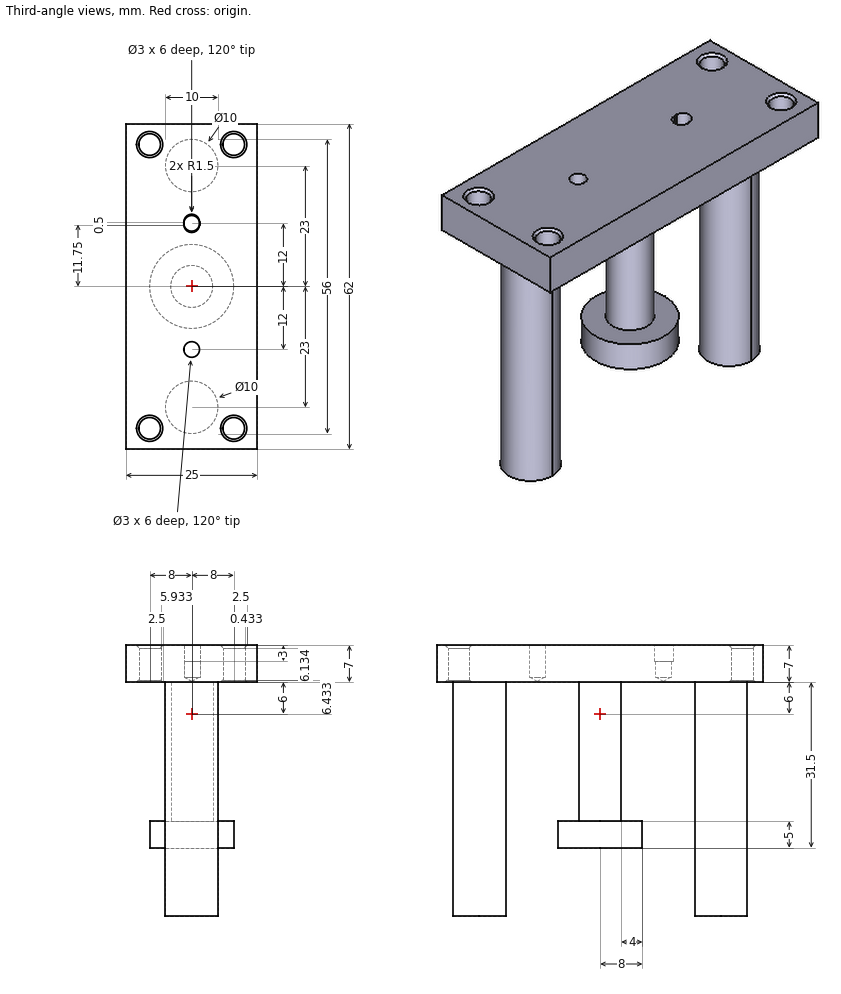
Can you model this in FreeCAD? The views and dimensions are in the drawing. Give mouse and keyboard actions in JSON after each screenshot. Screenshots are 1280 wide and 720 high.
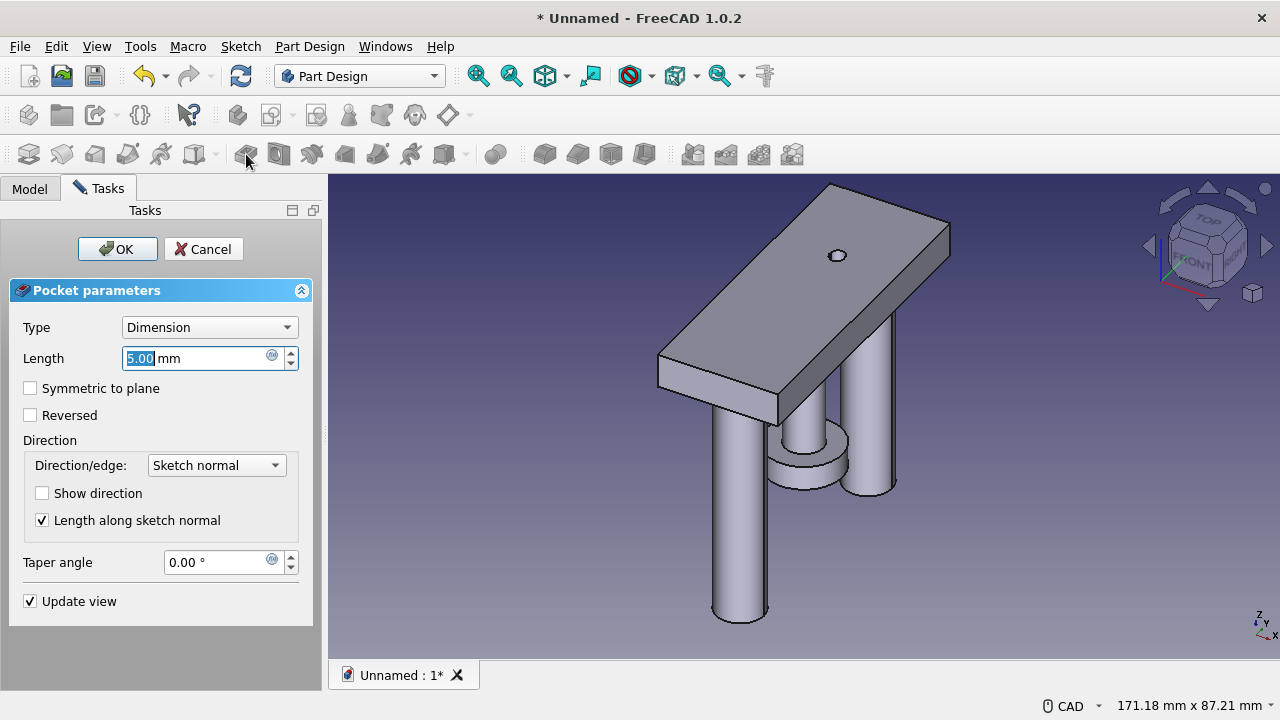
{"action": "type", "text": "3"}
{"action": "key", "text": "Tab"}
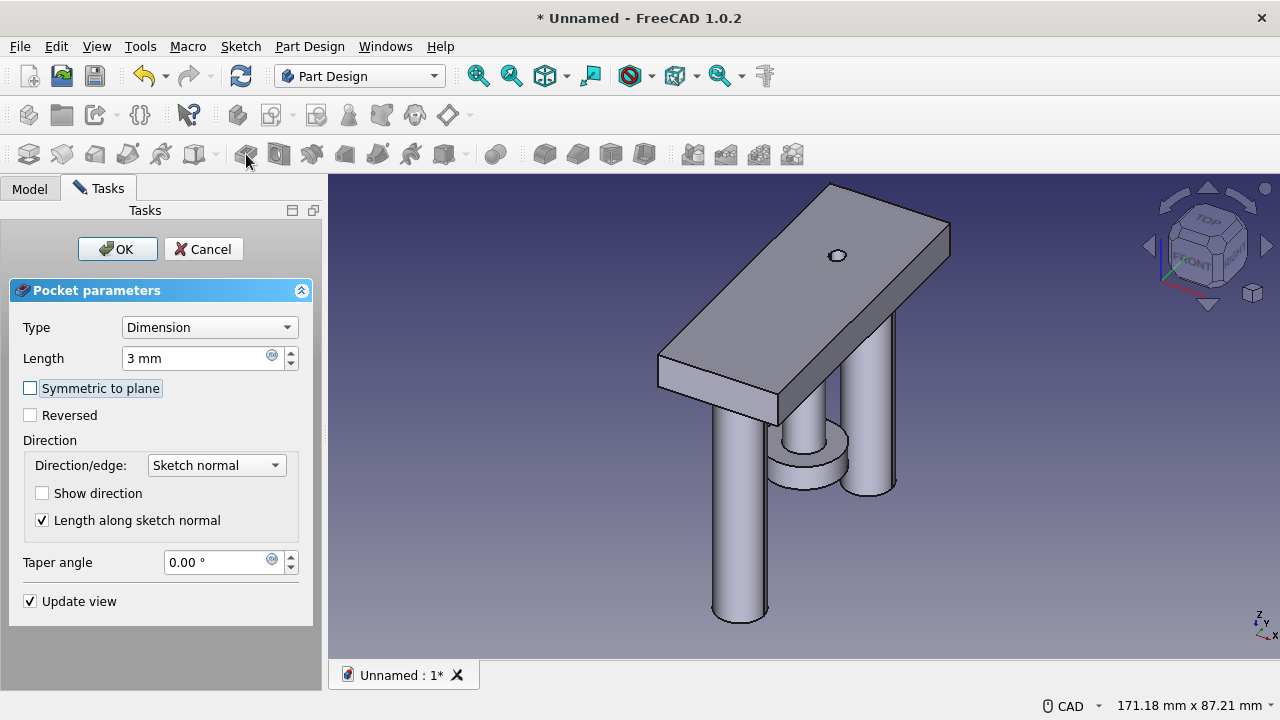
{"action": "left_click", "coordinate": [118, 249]}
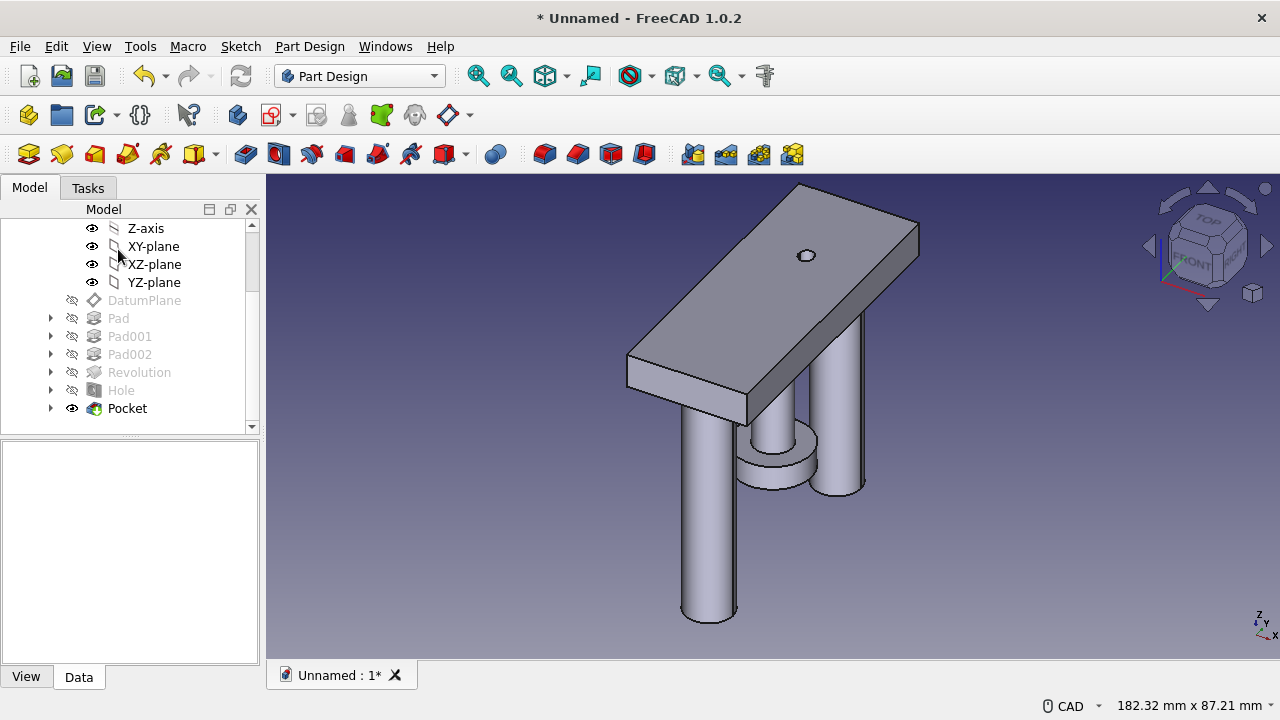
{"action": "left_click", "coordinate": [748, 312]}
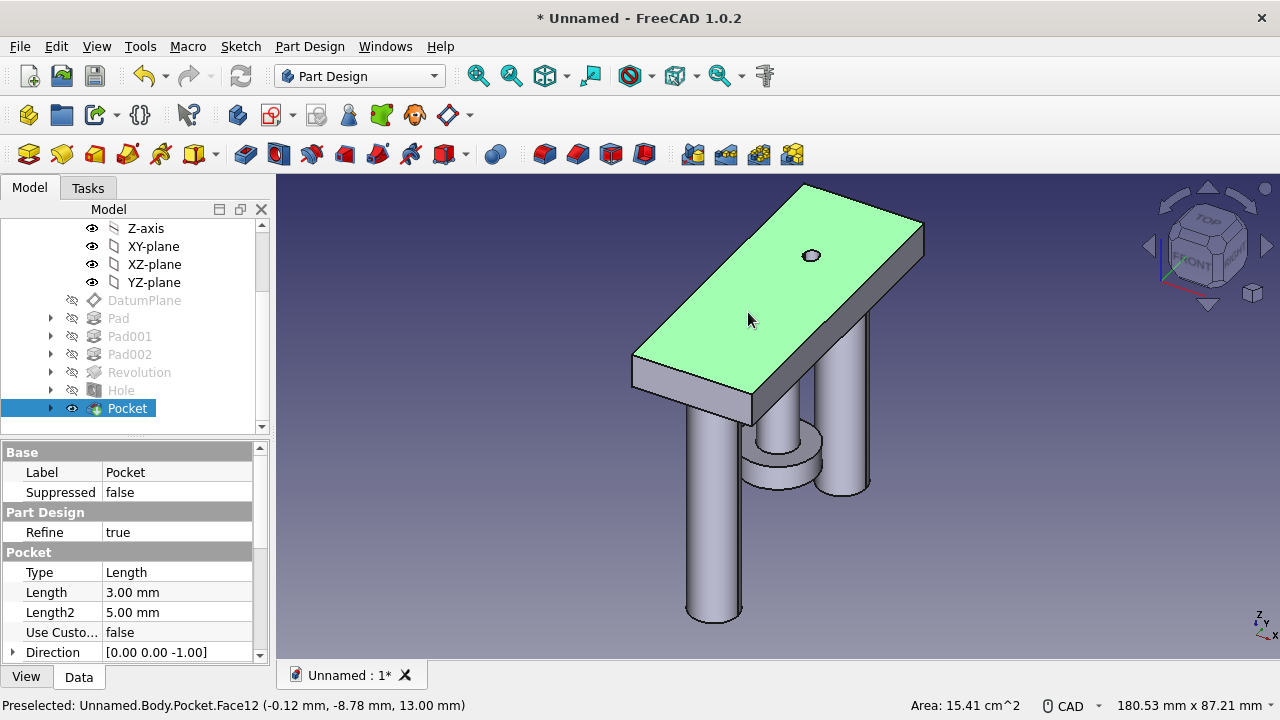
{"action": "left_click", "coordinate": [270, 116]}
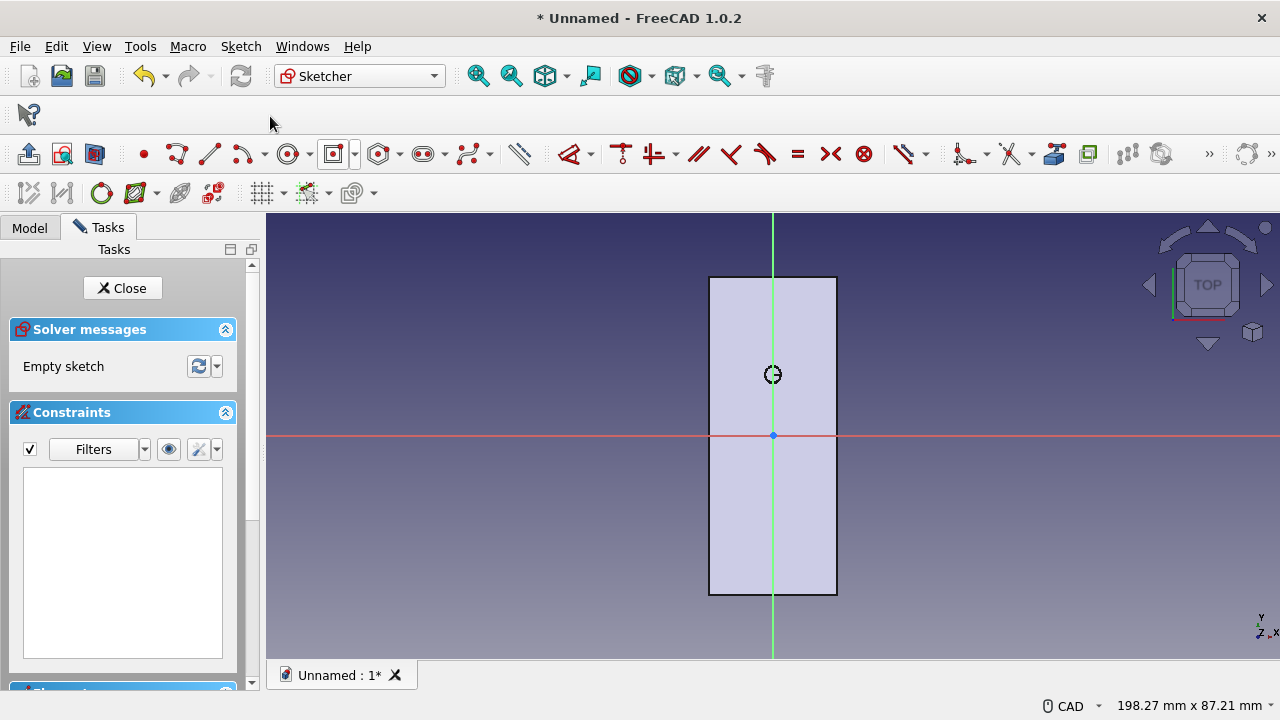
{"action": "scroll", "coordinate": [777, 501], "scroll_direction": "up", "scroll_amount": 14}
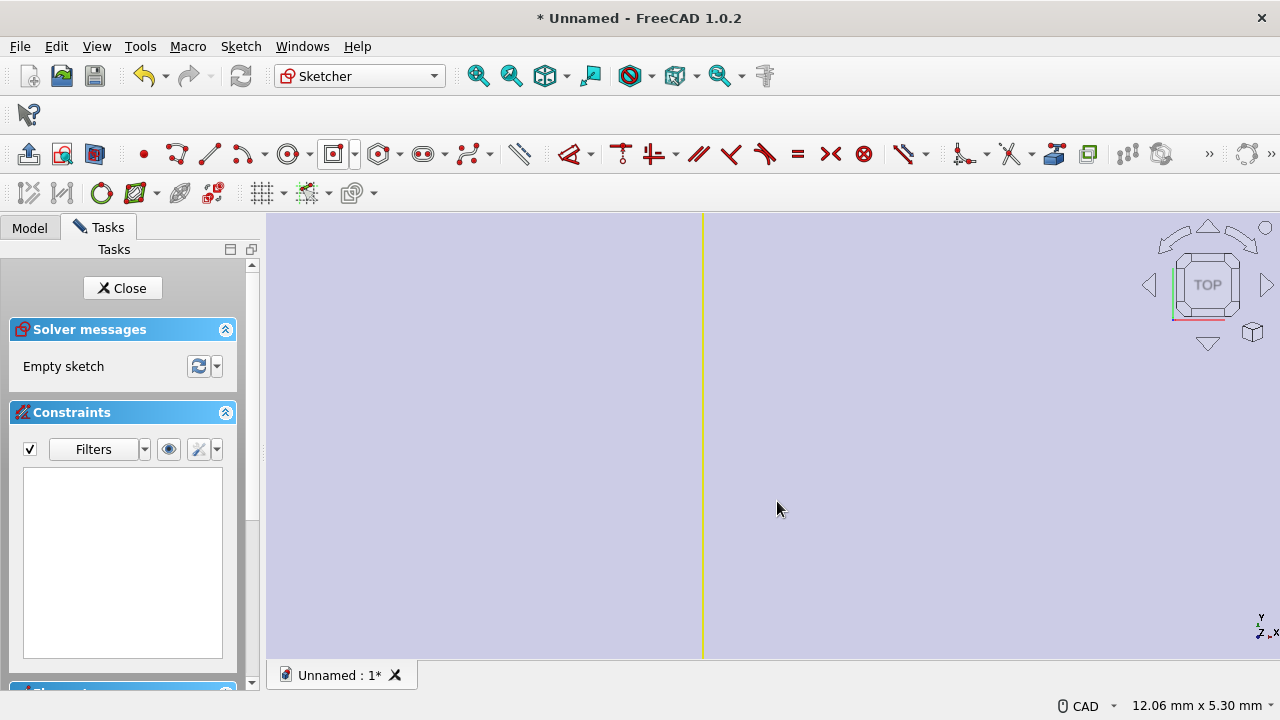
{"action": "left_click", "coordinate": [288, 154]}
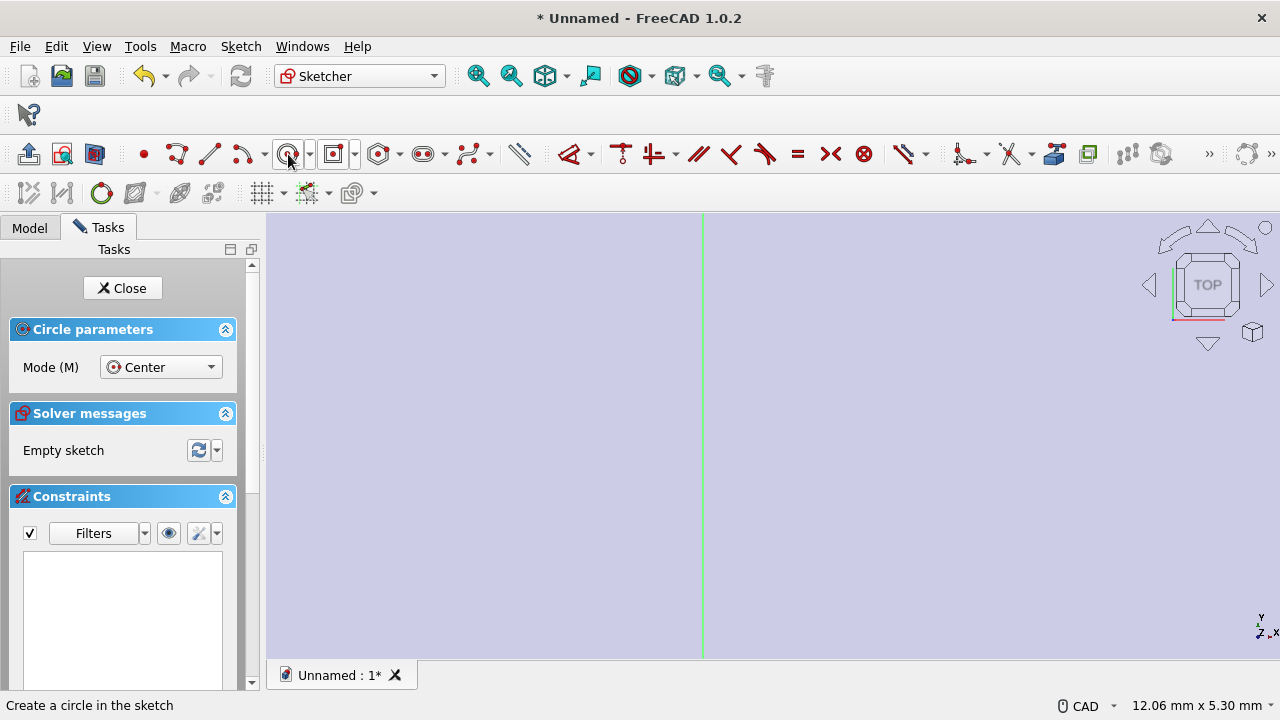
{"action": "left_click", "coordinate": [703, 431]}
{"action": "left_click", "coordinate": [793, 342]}
{"action": "key", "text": "Escape"}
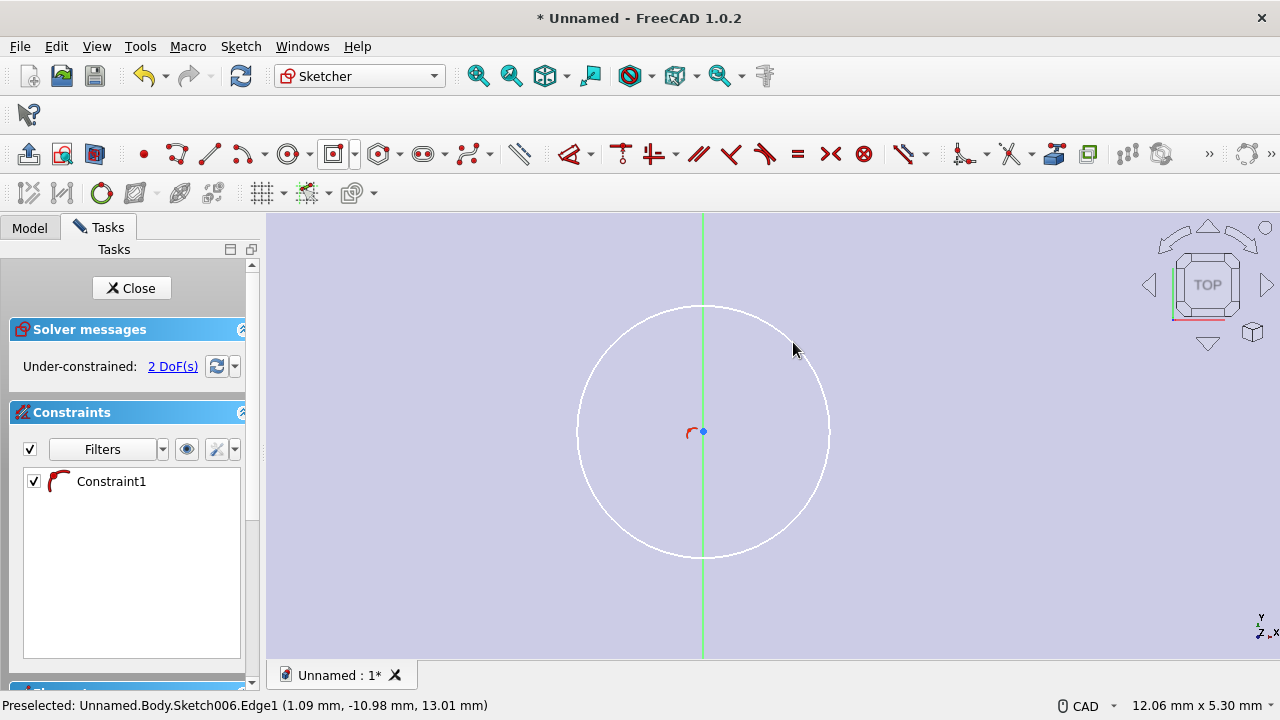
{"action": "left_click", "coordinate": [568, 154]}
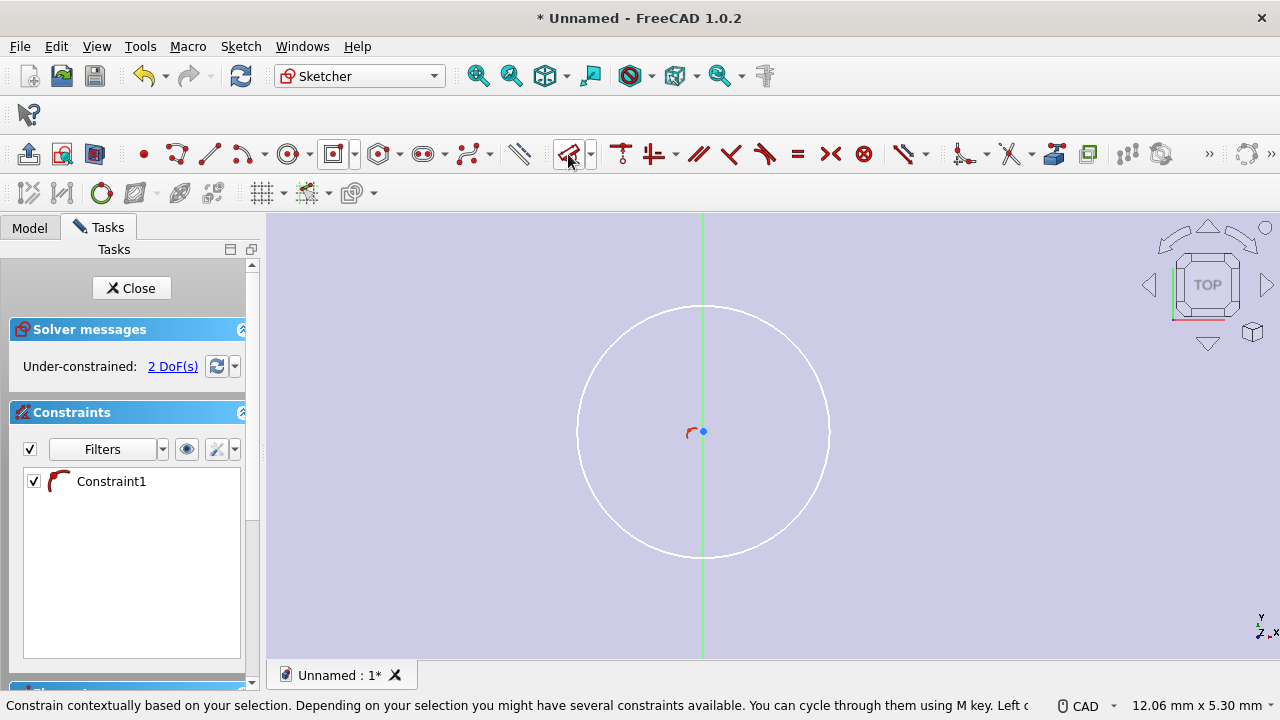
{"action": "left_click", "coordinate": [792, 342]}
{"action": "left_click", "coordinate": [814, 319]}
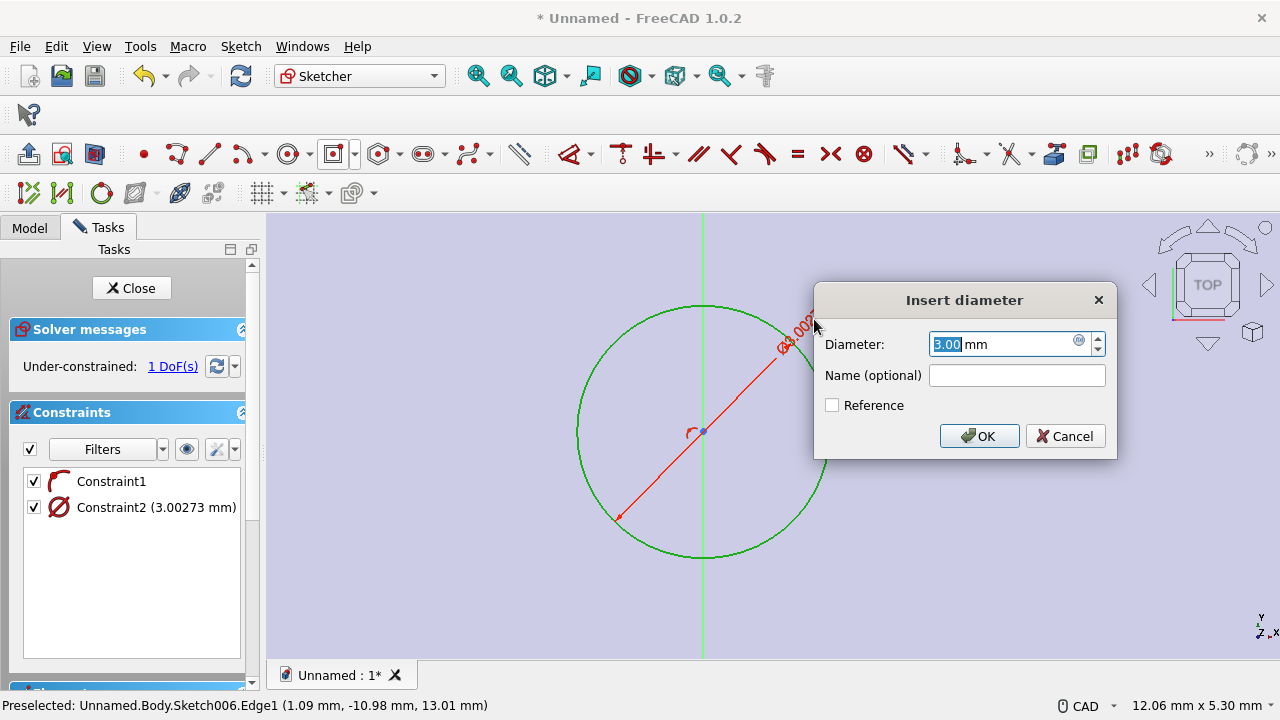
{"action": "type", "text": "3"}
{"action": "key", "text": "Return"}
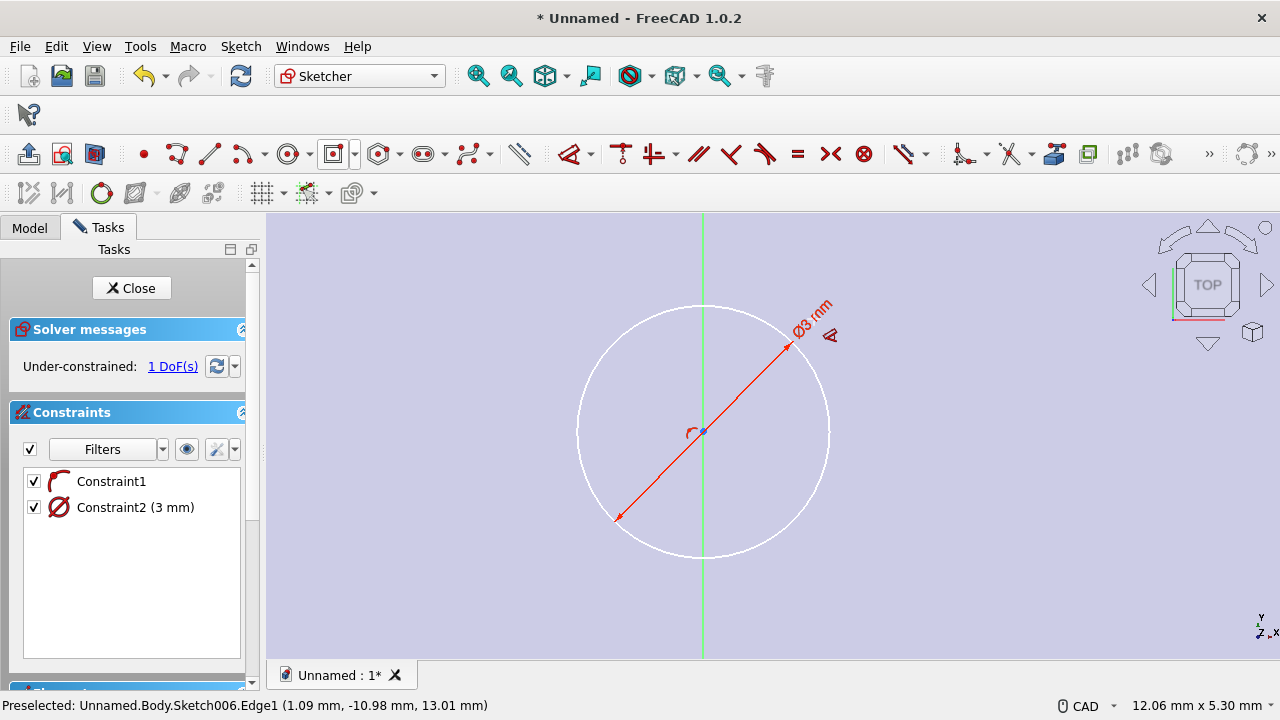
{"action": "left_click", "coordinate": [703, 432]}
{"action": "left_click", "coordinate": [737, 337]}